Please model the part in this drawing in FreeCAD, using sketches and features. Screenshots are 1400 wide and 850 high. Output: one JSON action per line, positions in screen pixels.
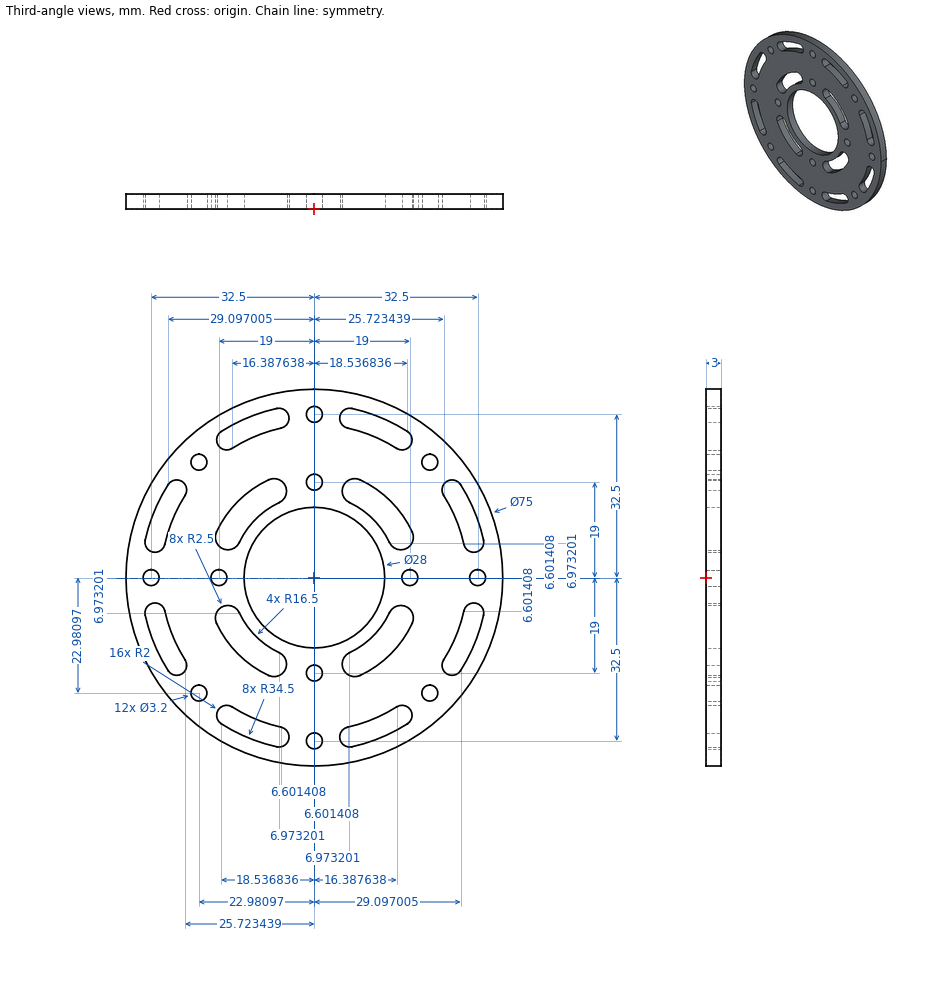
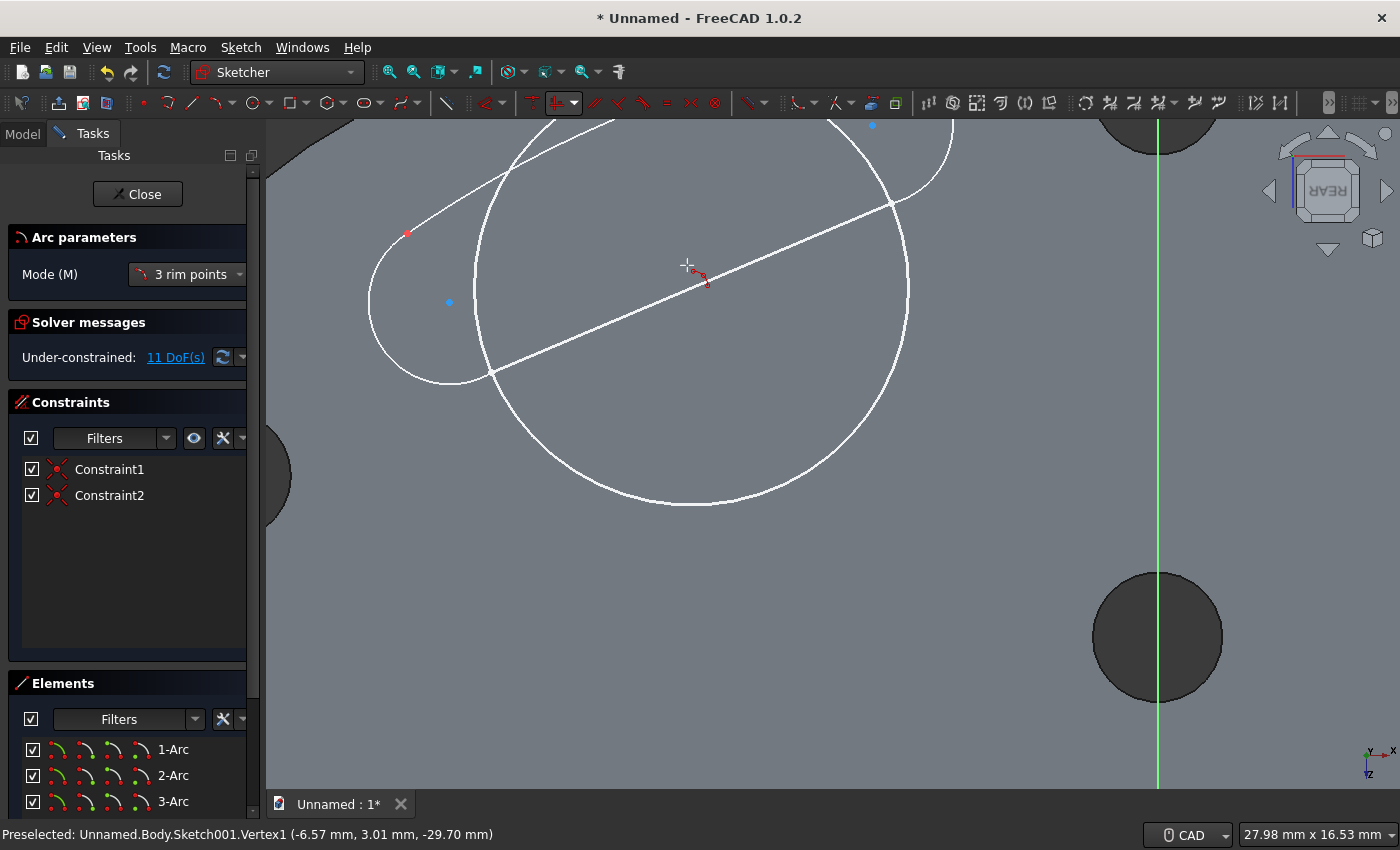
{"action": "left_click", "coordinate": [685, 265]}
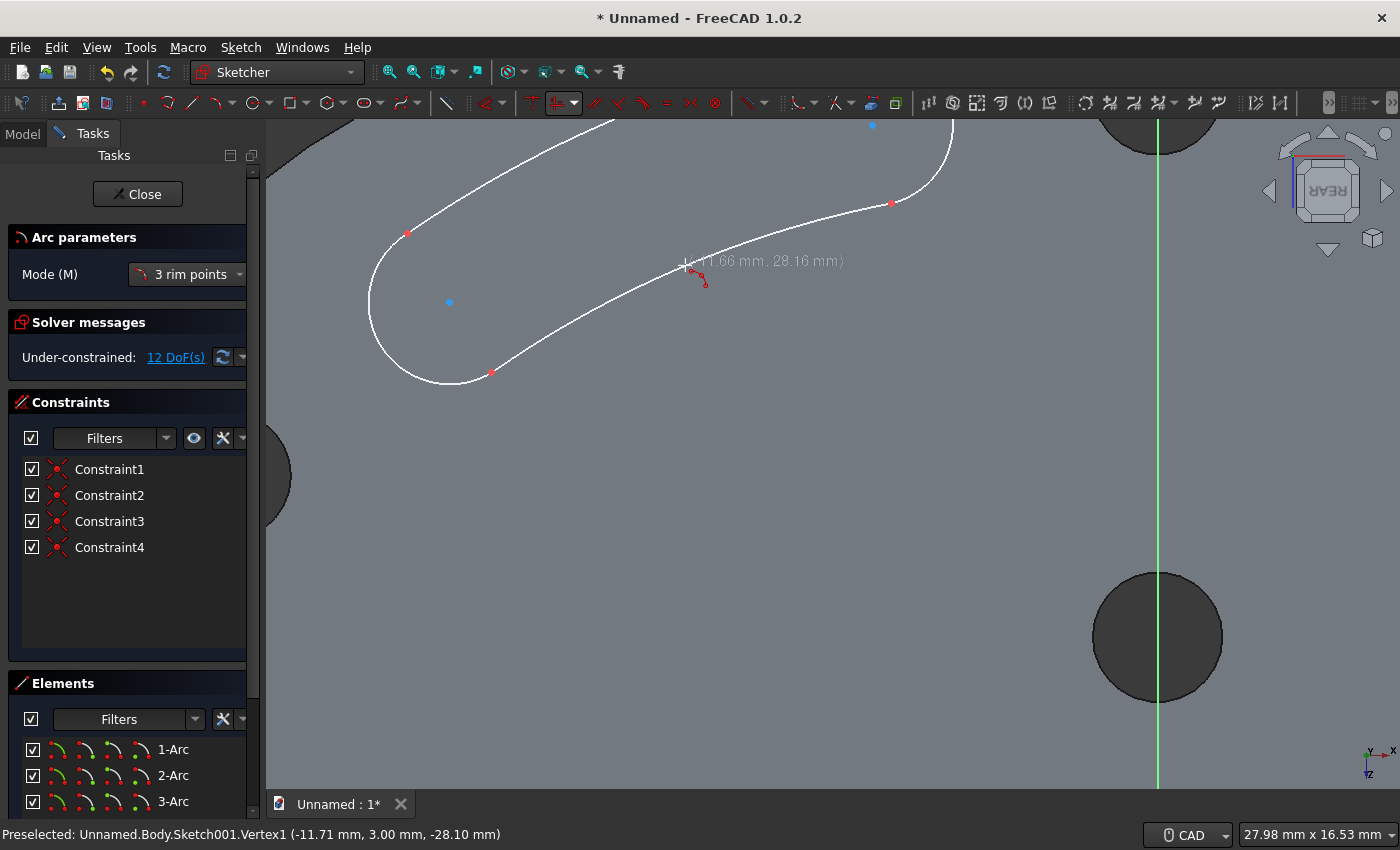
{"action": "scroll", "coordinate": [687, 265], "scroll_direction": "down", "scroll_amount": 9}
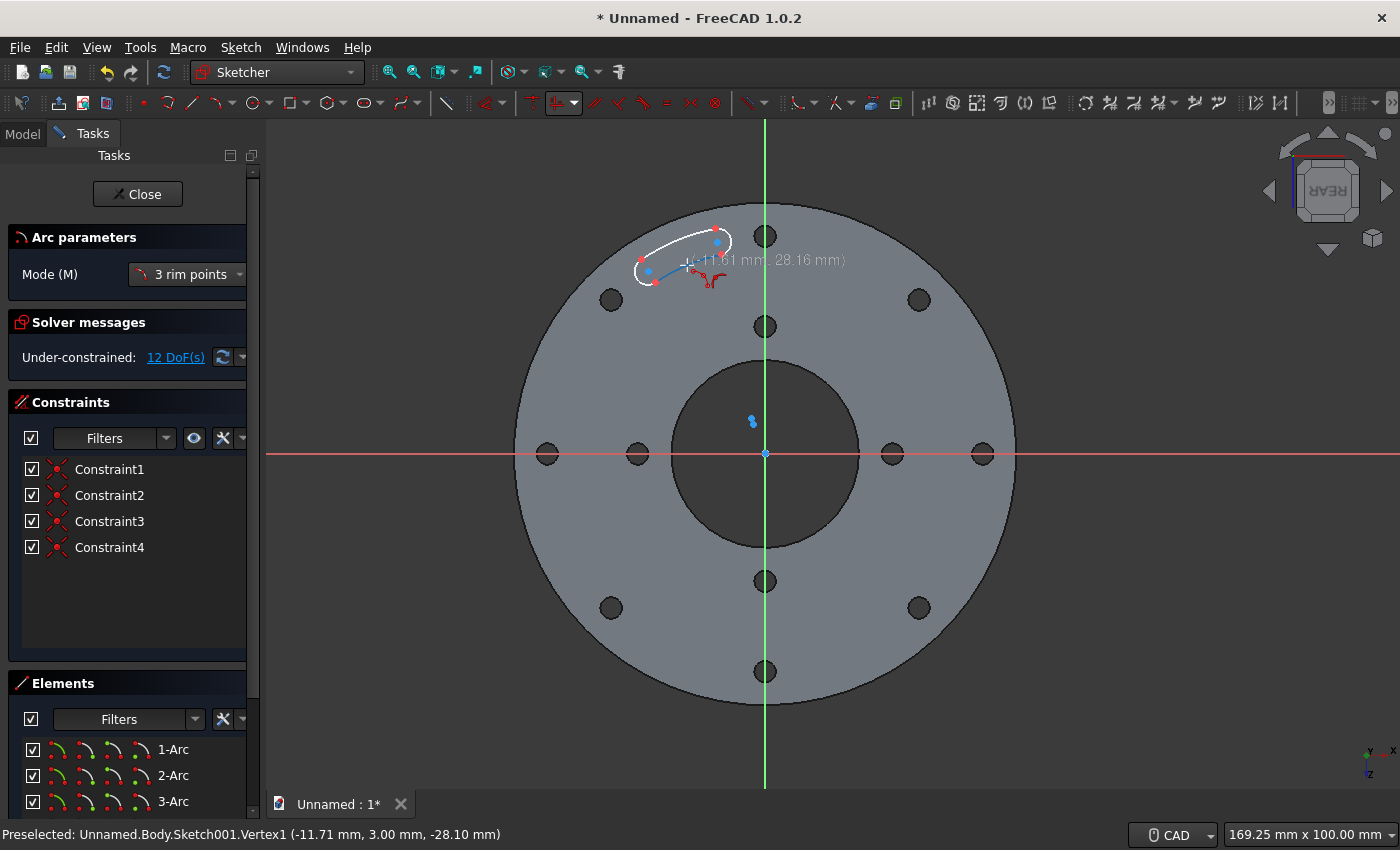
{"action": "left_click", "coordinate": [665, 407]}
{"action": "left_click", "coordinate": [718, 354]}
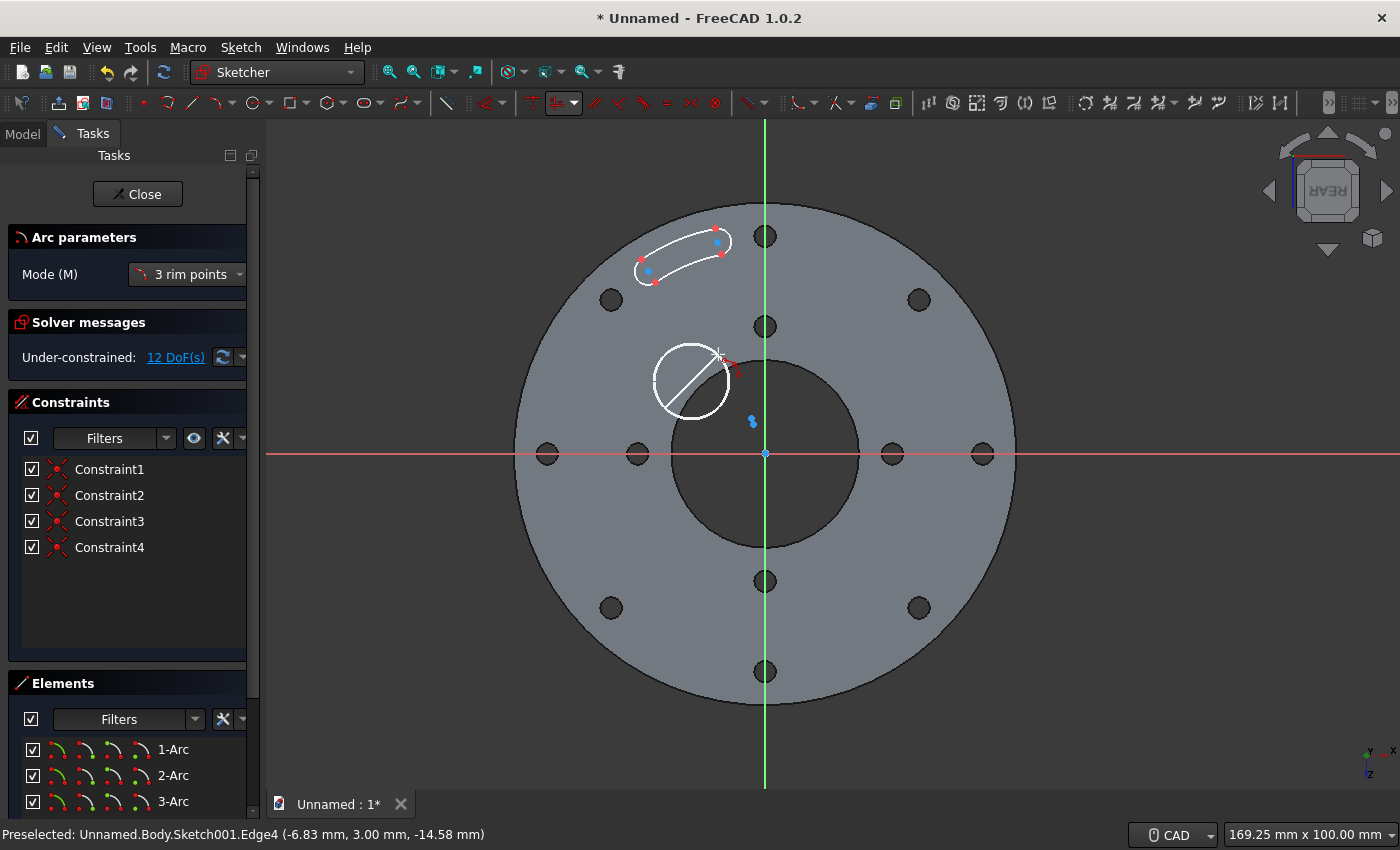
{"action": "scroll", "coordinate": [687, 376], "scroll_direction": "up", "scroll_amount": 5}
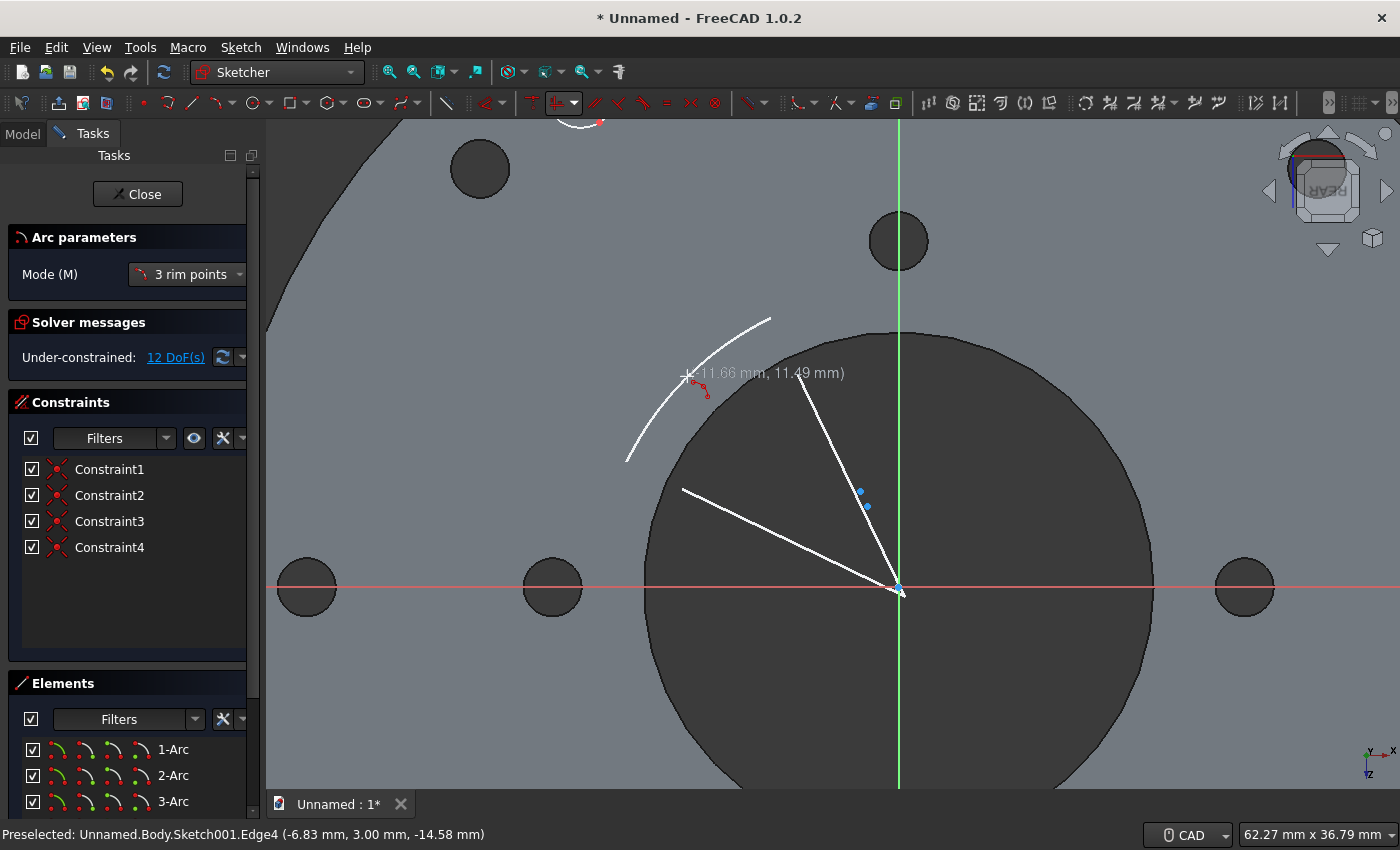
{"action": "left_click", "coordinate": [686, 375]}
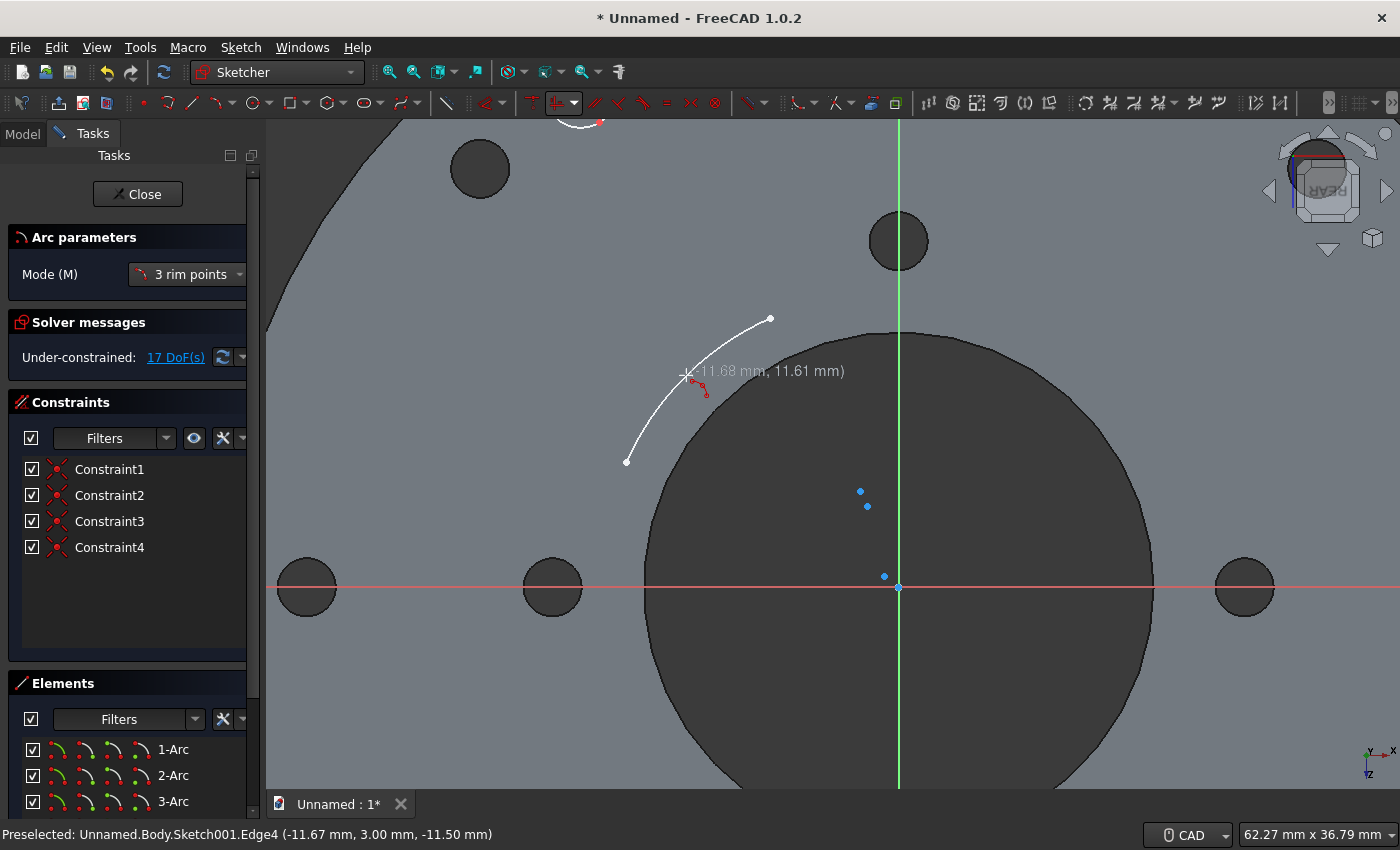
{"action": "left_click", "coordinate": [771, 318]}
{"action": "left_click", "coordinate": [733, 232]}
{"action": "left_click", "coordinate": [794, 255]}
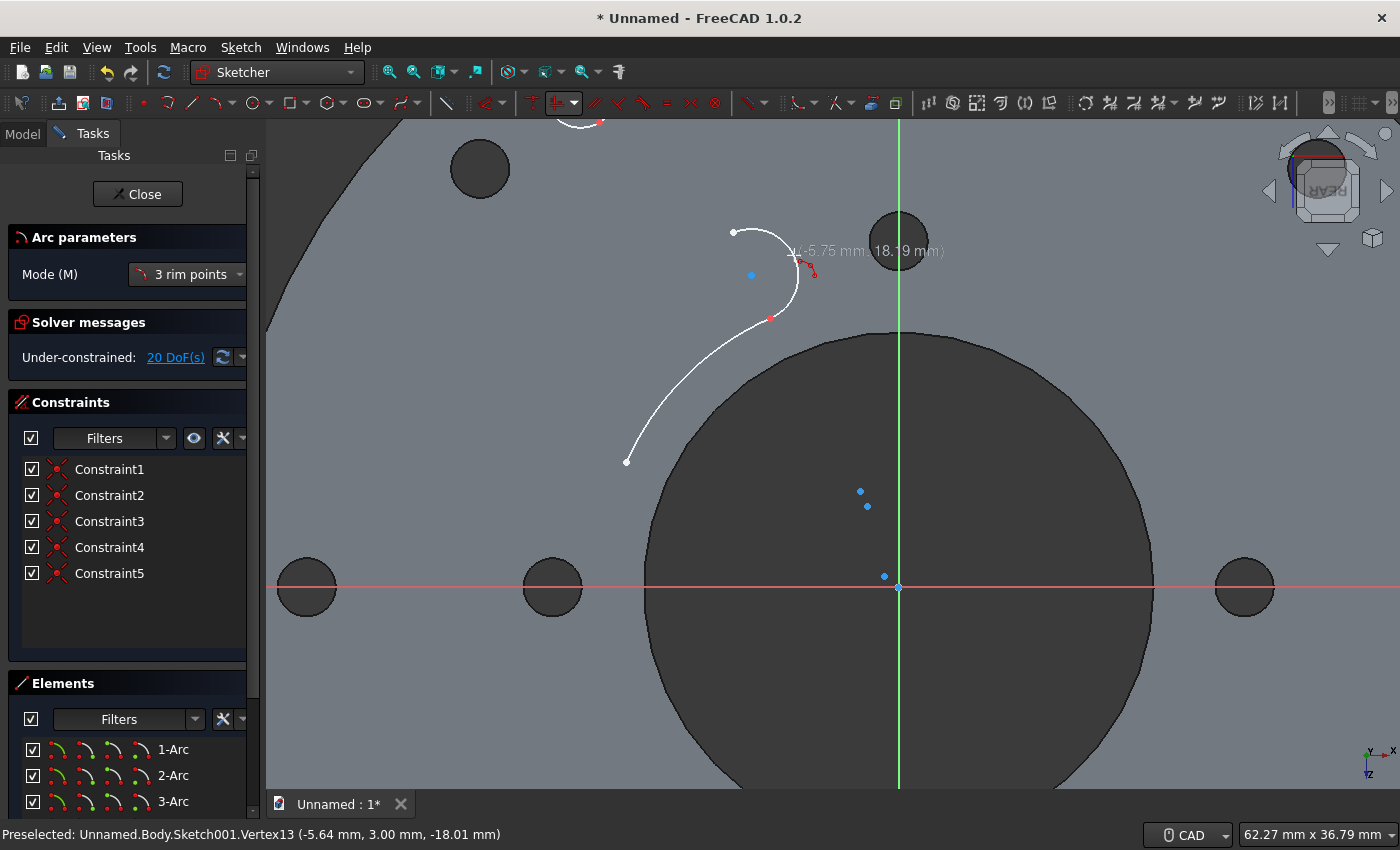
{"action": "left_click", "coordinate": [733, 233]}
{"action": "left_click", "coordinate": [544, 422]}
{"action": "left_click", "coordinate": [622, 310]}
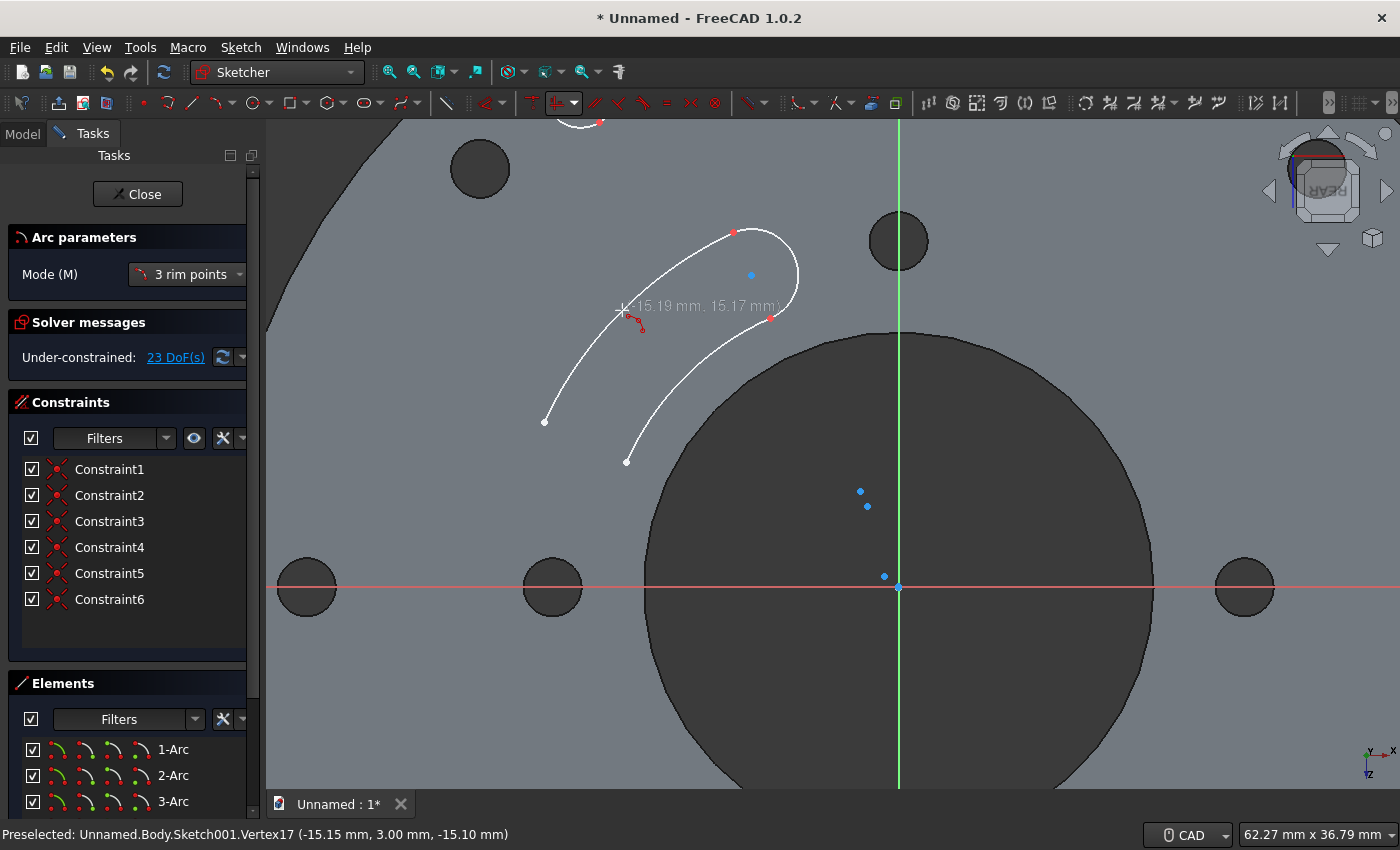
{"action": "left_click", "coordinate": [544, 423]}
{"action": "left_click", "coordinate": [627, 462]}
{"action": "left_click", "coordinate": [566, 482]}